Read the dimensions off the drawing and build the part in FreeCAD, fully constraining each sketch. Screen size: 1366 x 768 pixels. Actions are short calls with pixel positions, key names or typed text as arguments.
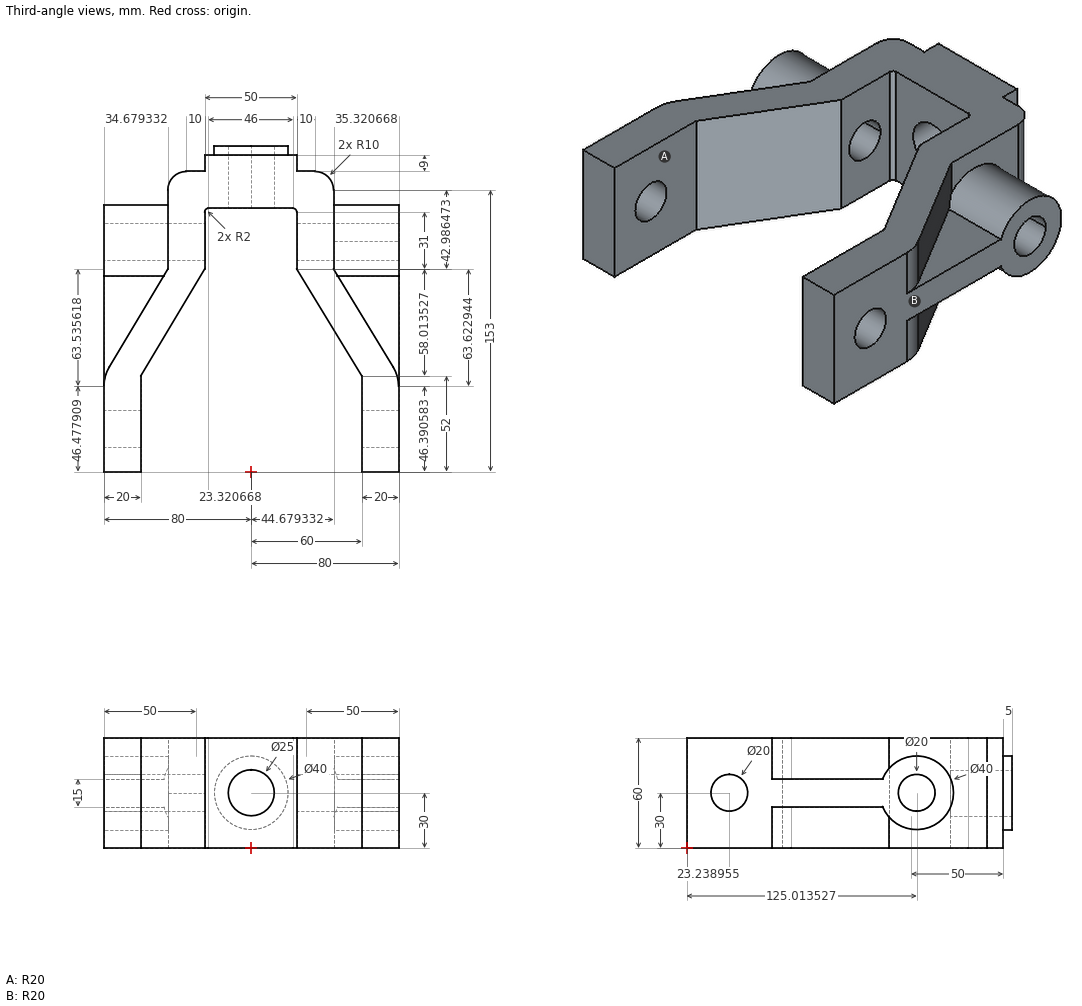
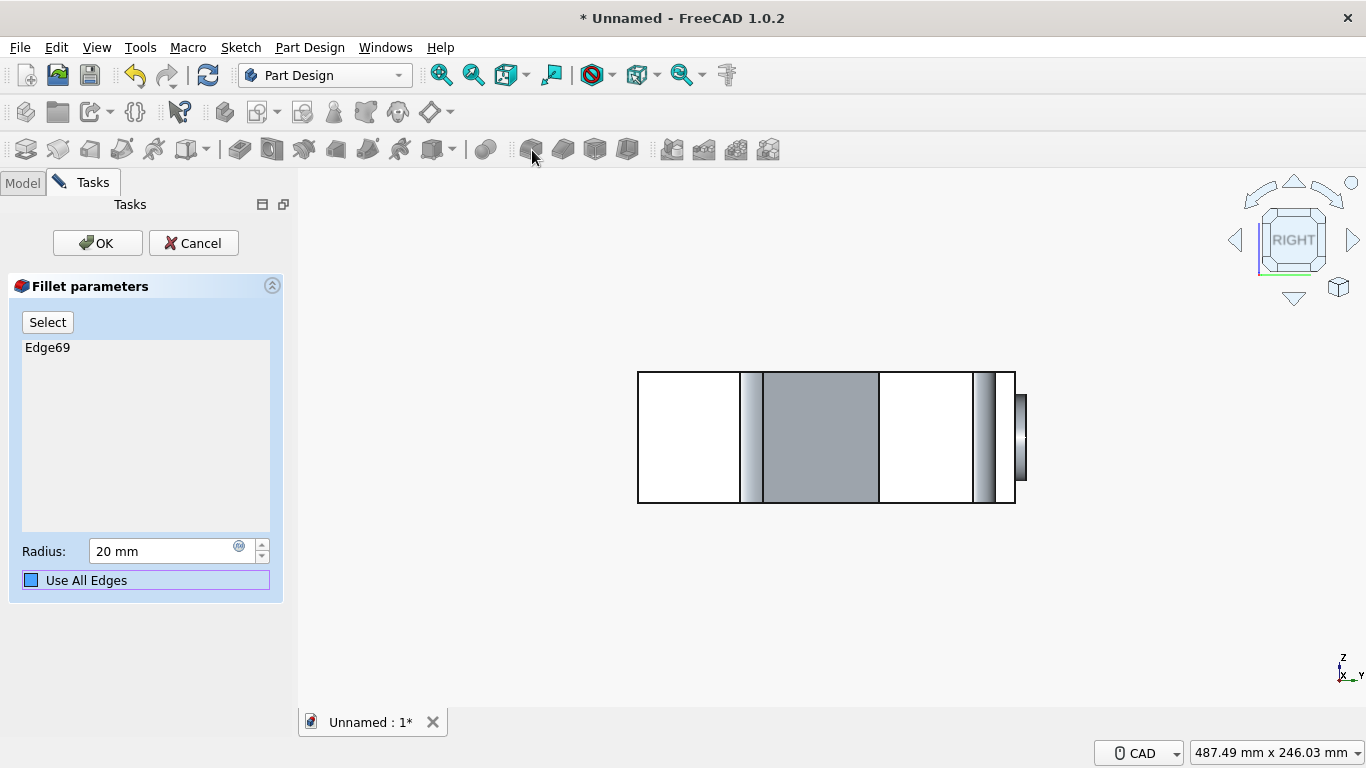
click(98, 243)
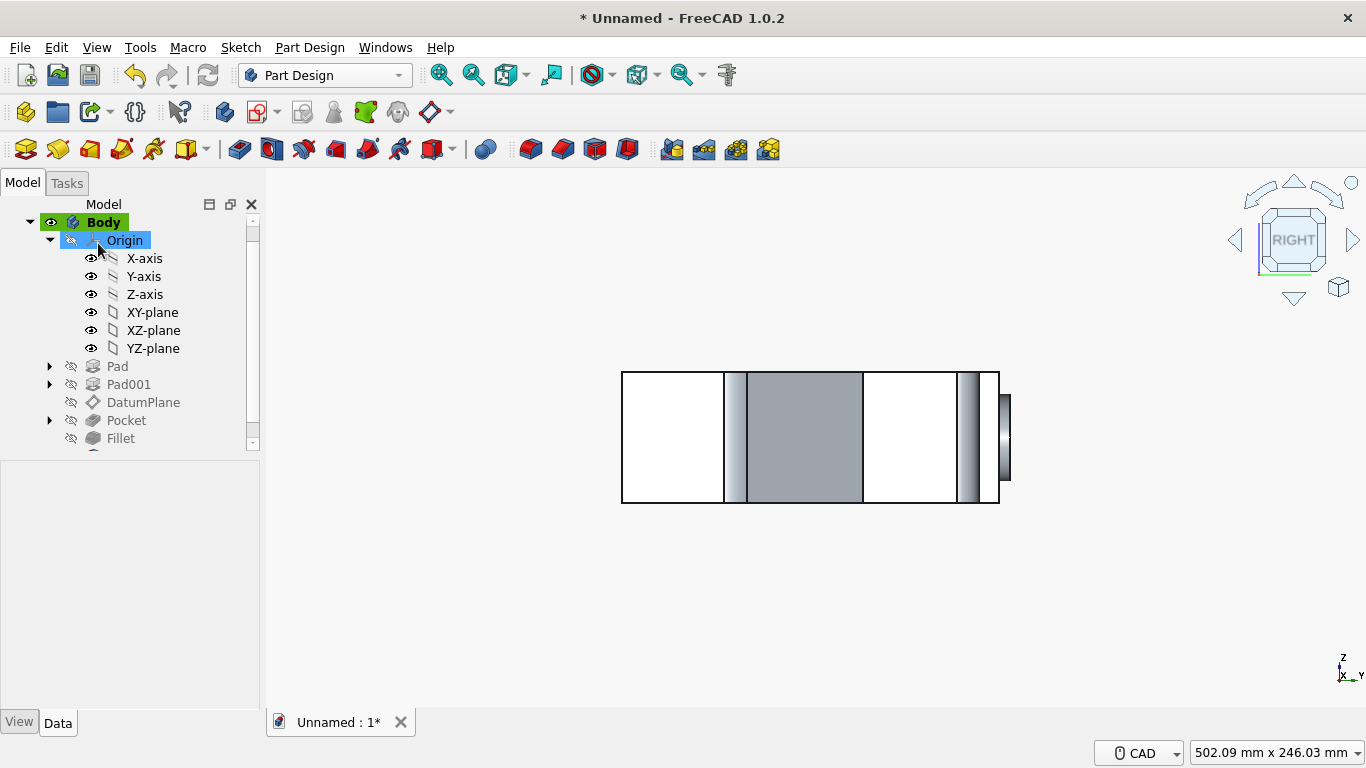
key(v)
key(f)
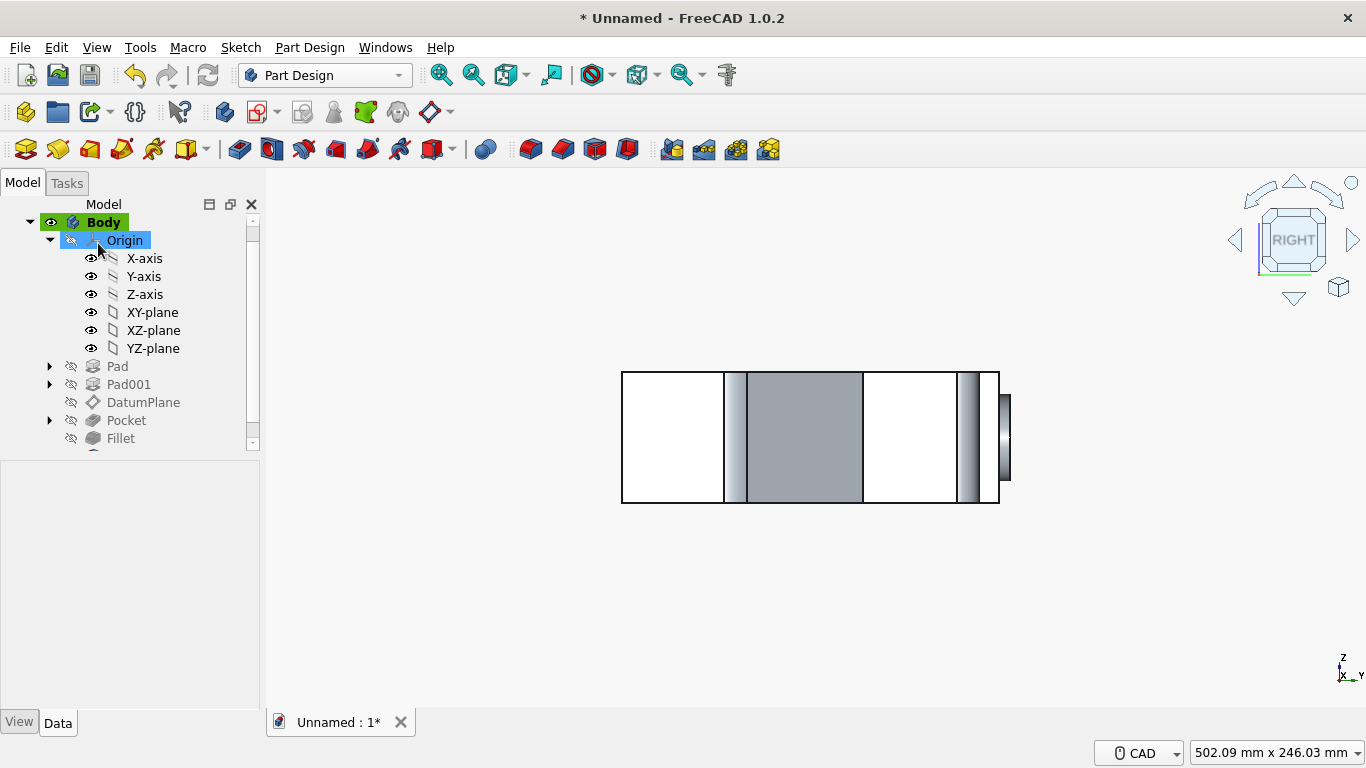
key(6)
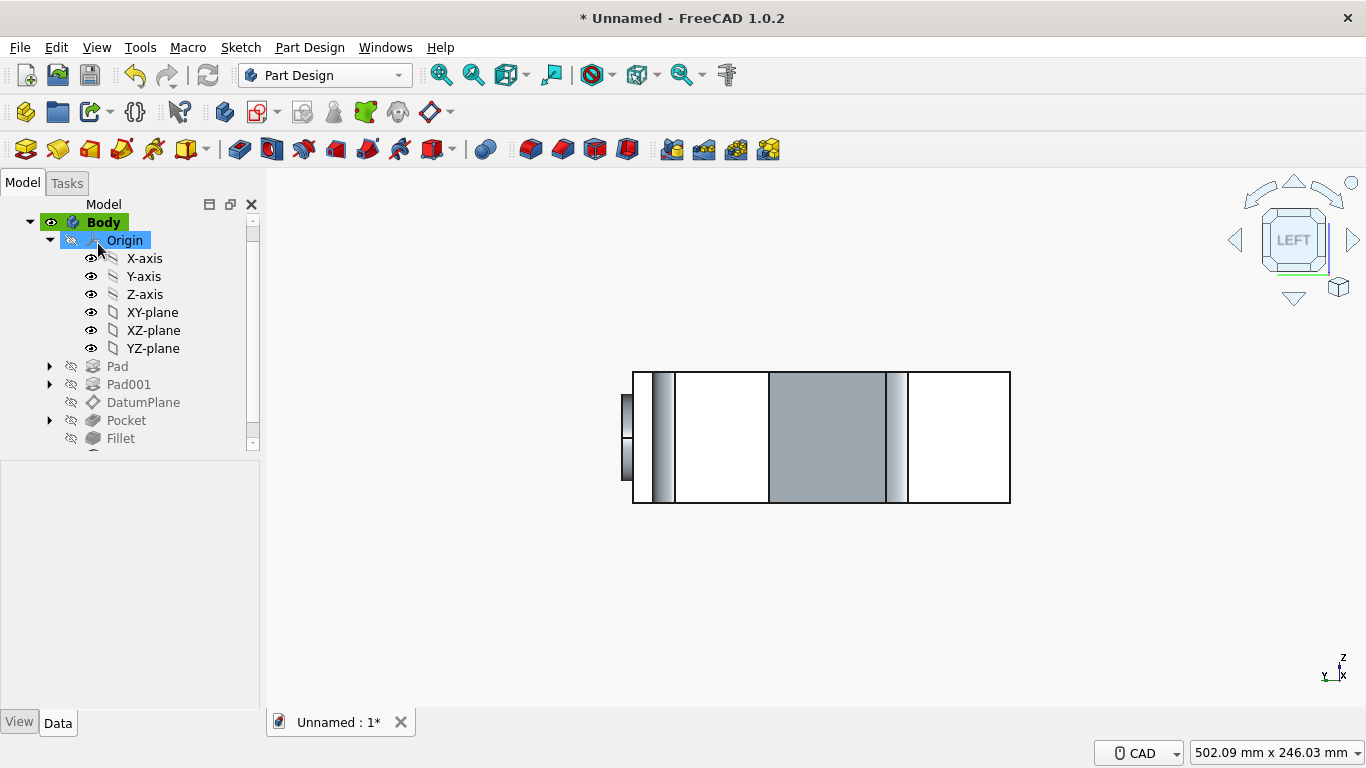
key(v)
key(f)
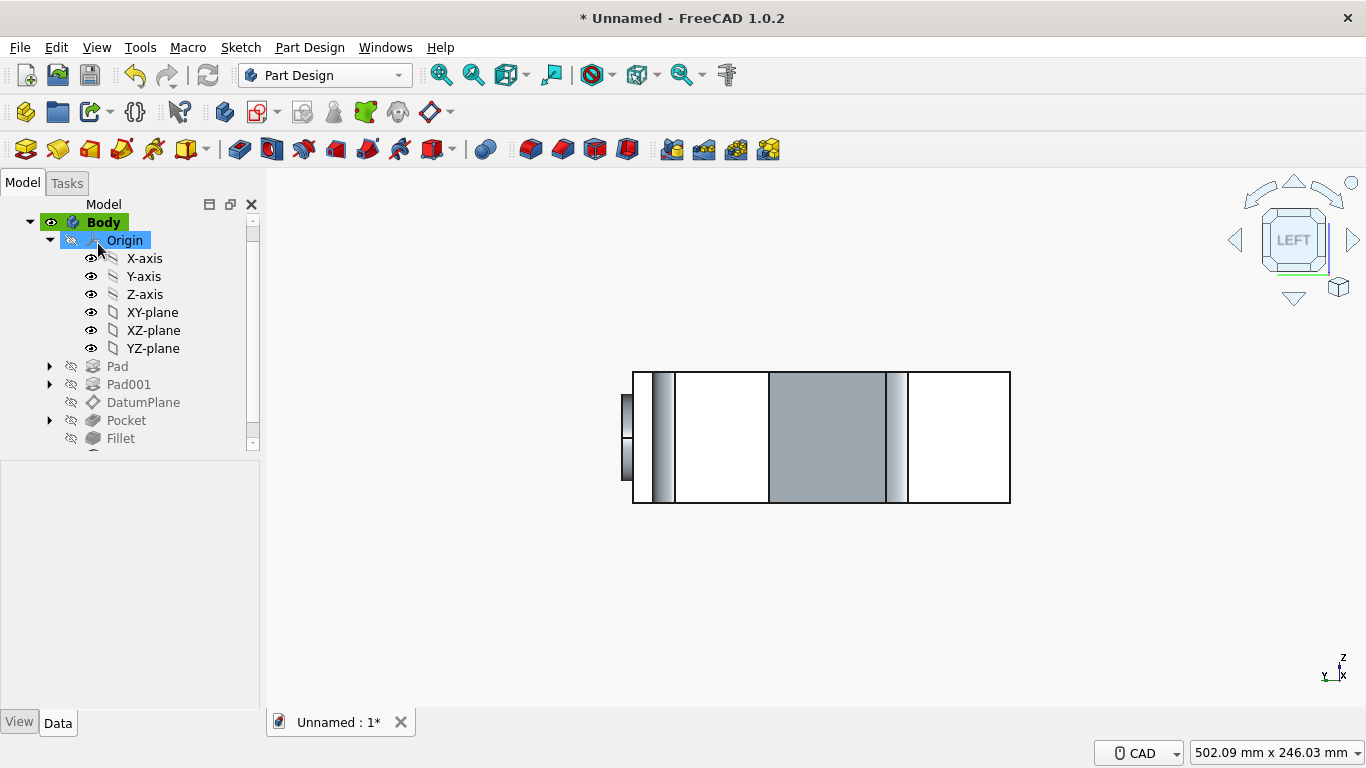
click(959, 436)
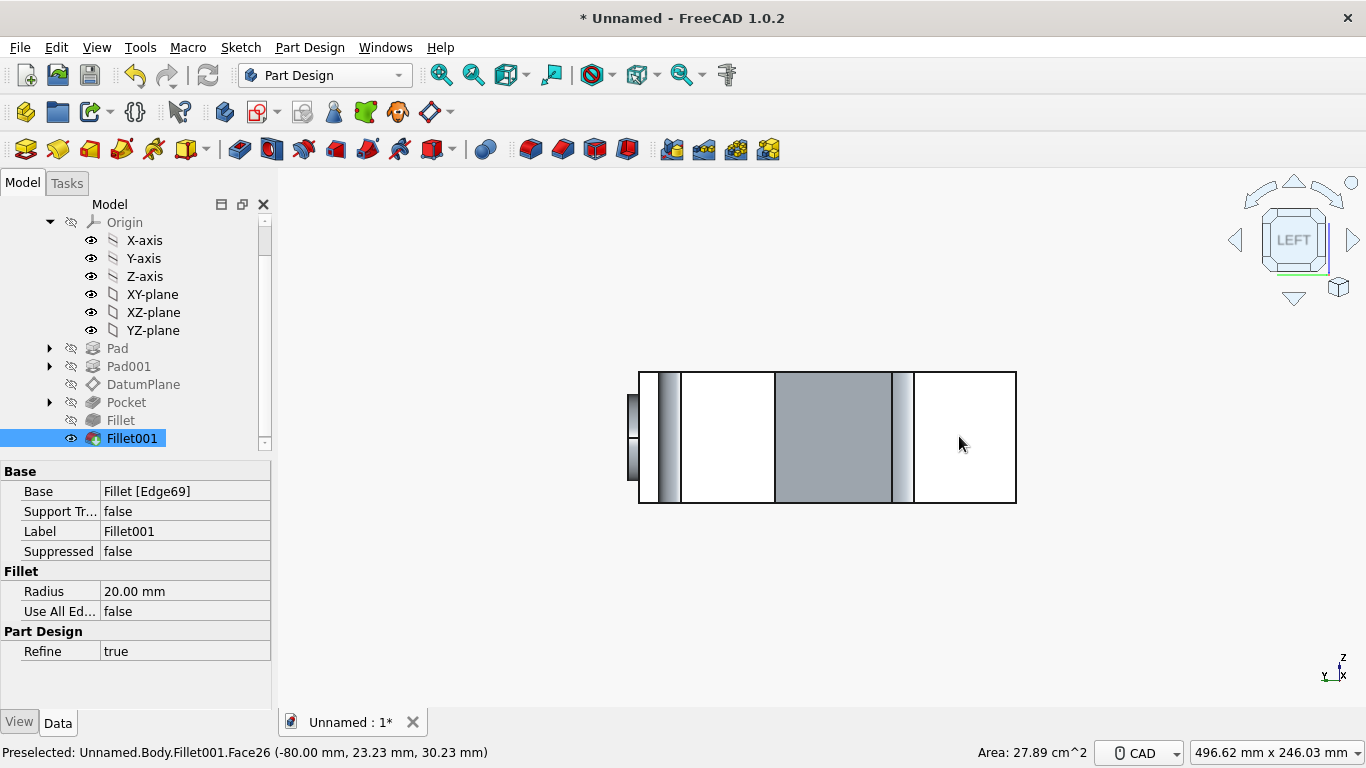
click(258, 112)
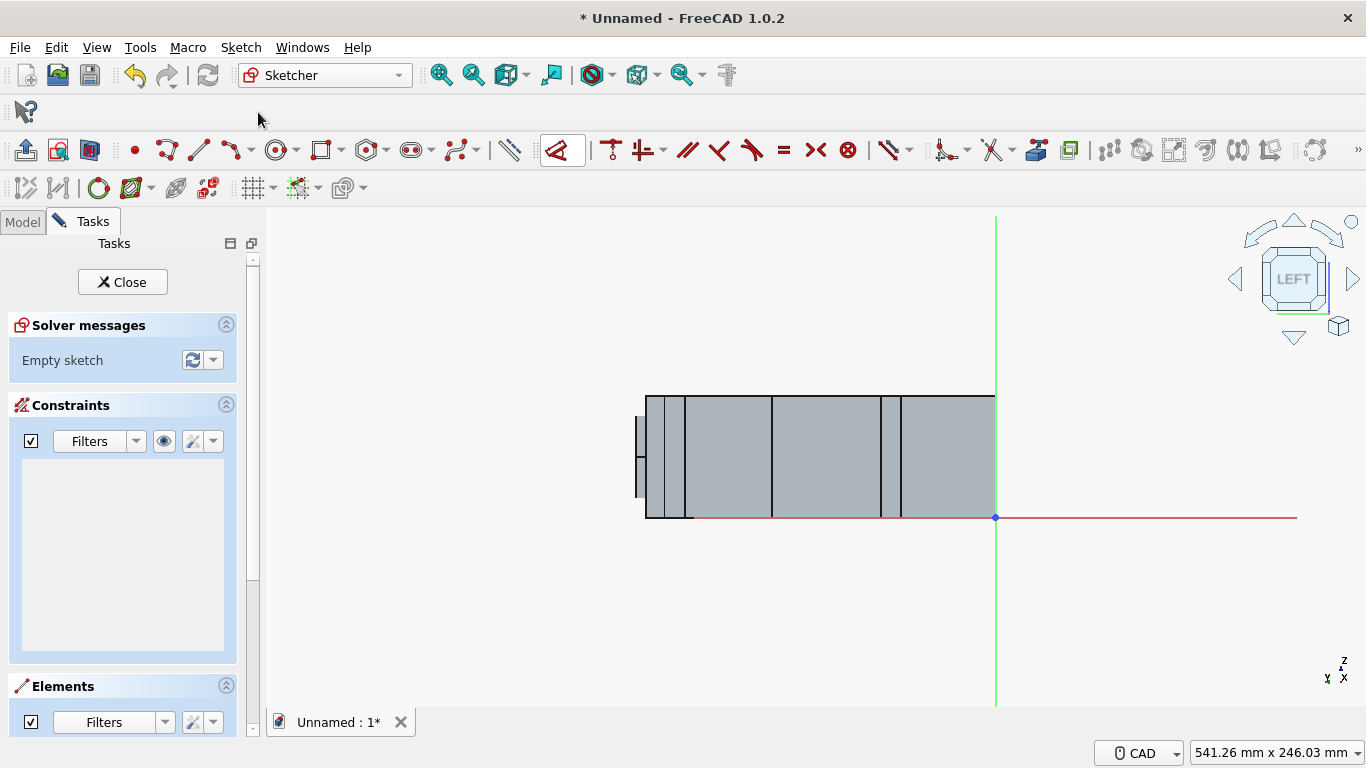
scroll(1032, 484, up, 7)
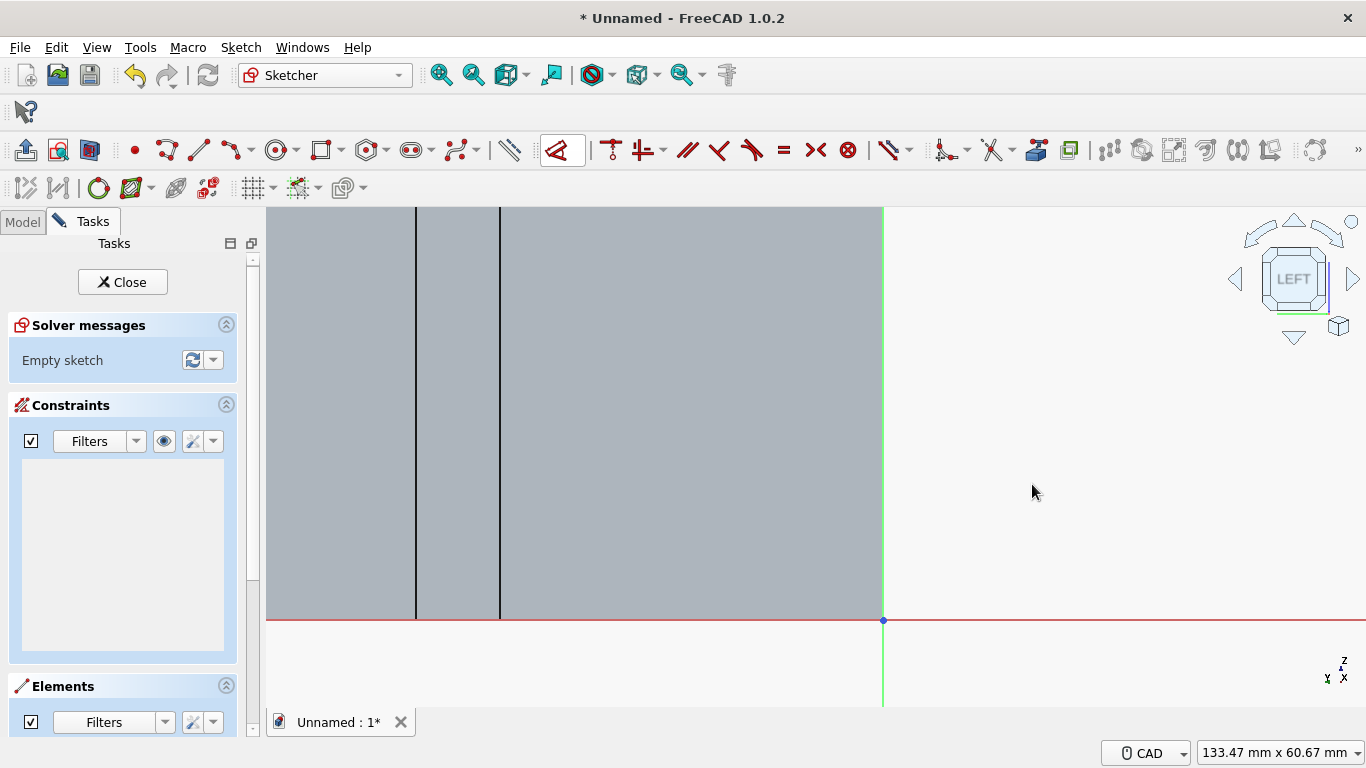
key(g)
key(c)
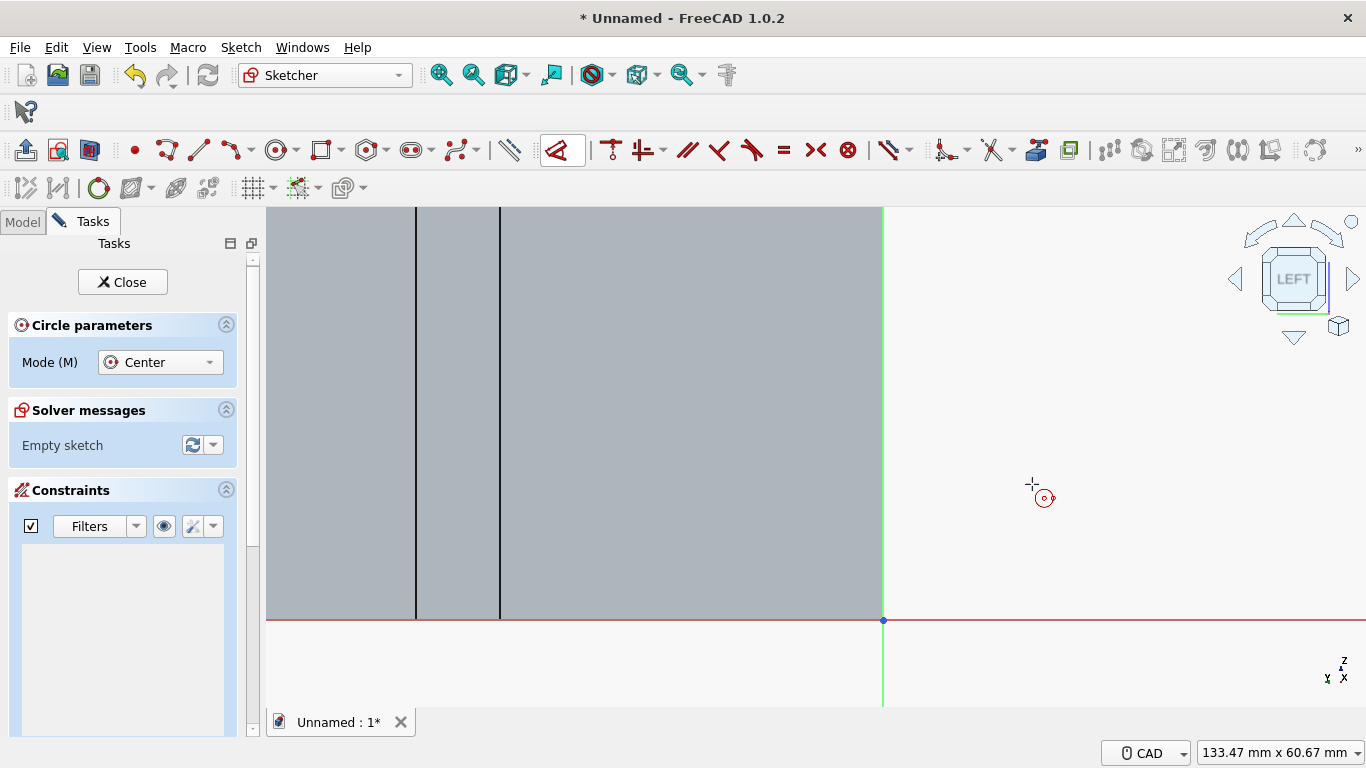
click(692, 373)
click(750, 315)
key(Escape)